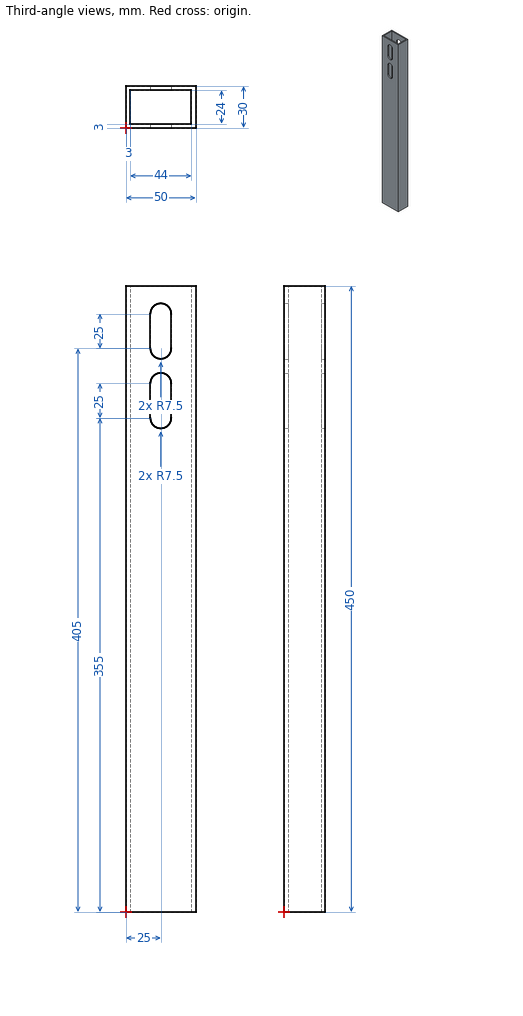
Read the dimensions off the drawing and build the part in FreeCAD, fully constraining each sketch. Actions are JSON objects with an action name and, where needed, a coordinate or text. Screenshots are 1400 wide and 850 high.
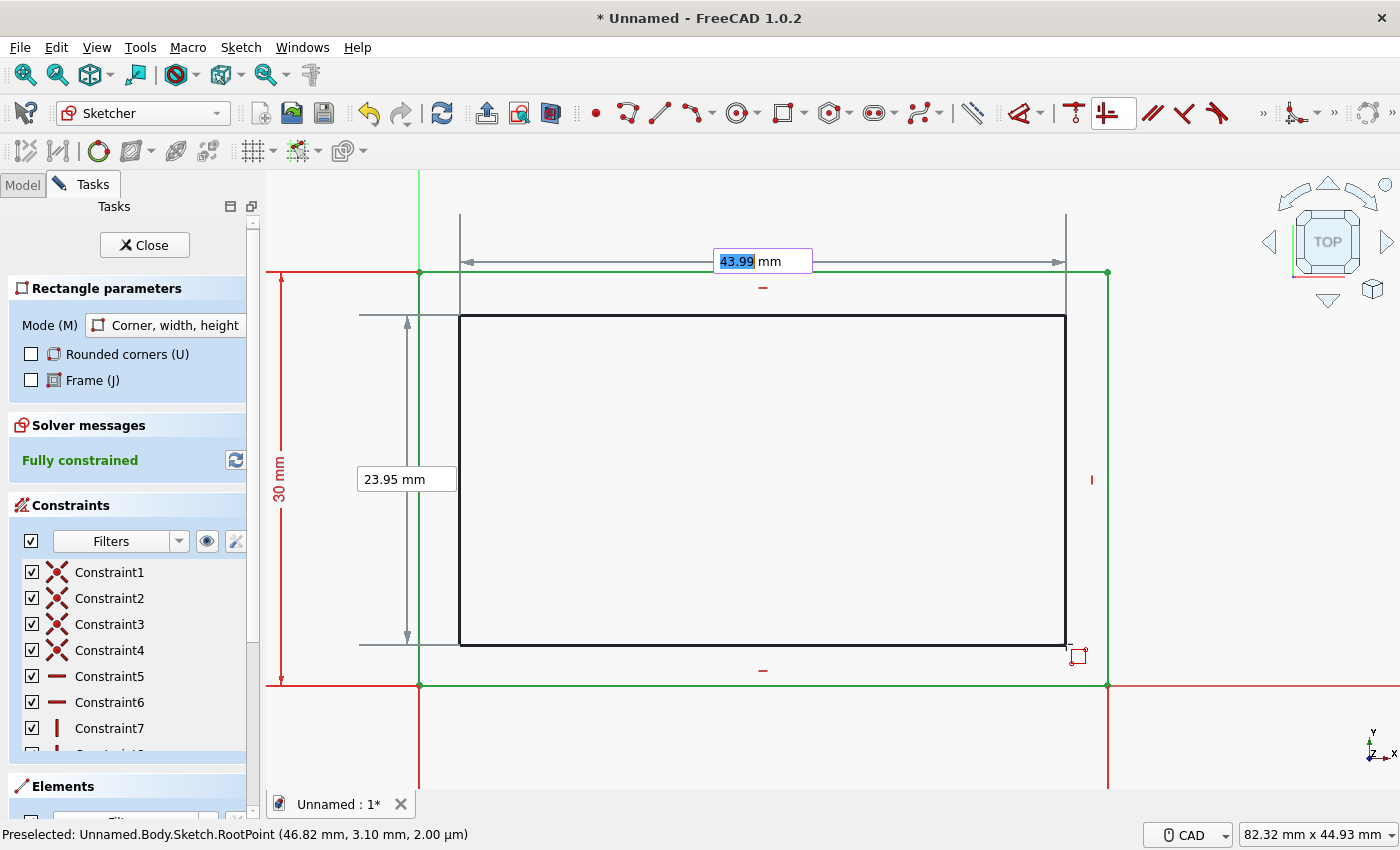
{"action": "type", "text": "44"}
{"action": "key", "text": "Tab"}
{"action": "type", "text": "24"}
{"action": "key", "text": "Return"}
{"action": "key", "text": "Escape"}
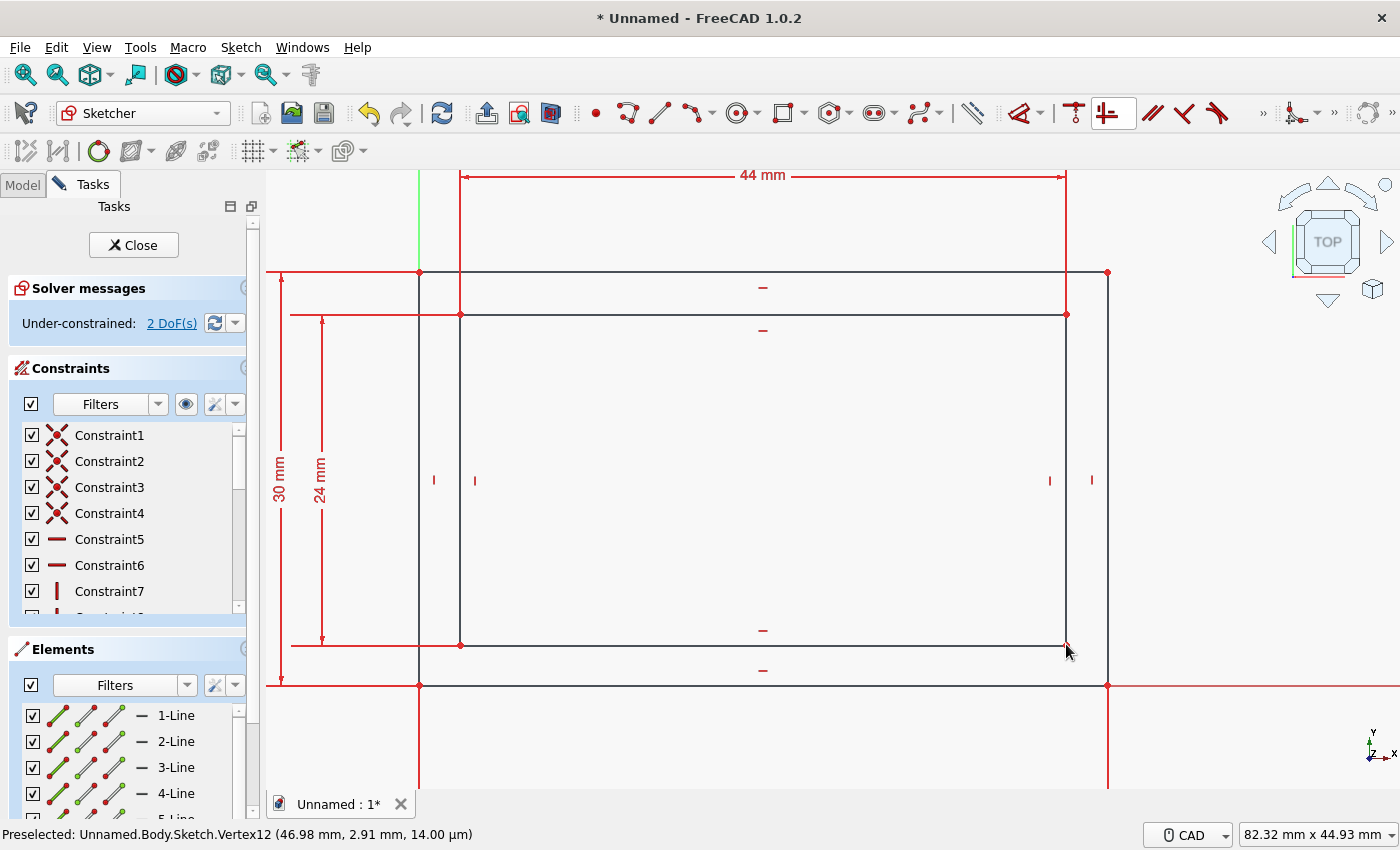
{"action": "left_click", "coordinate": [460, 315]}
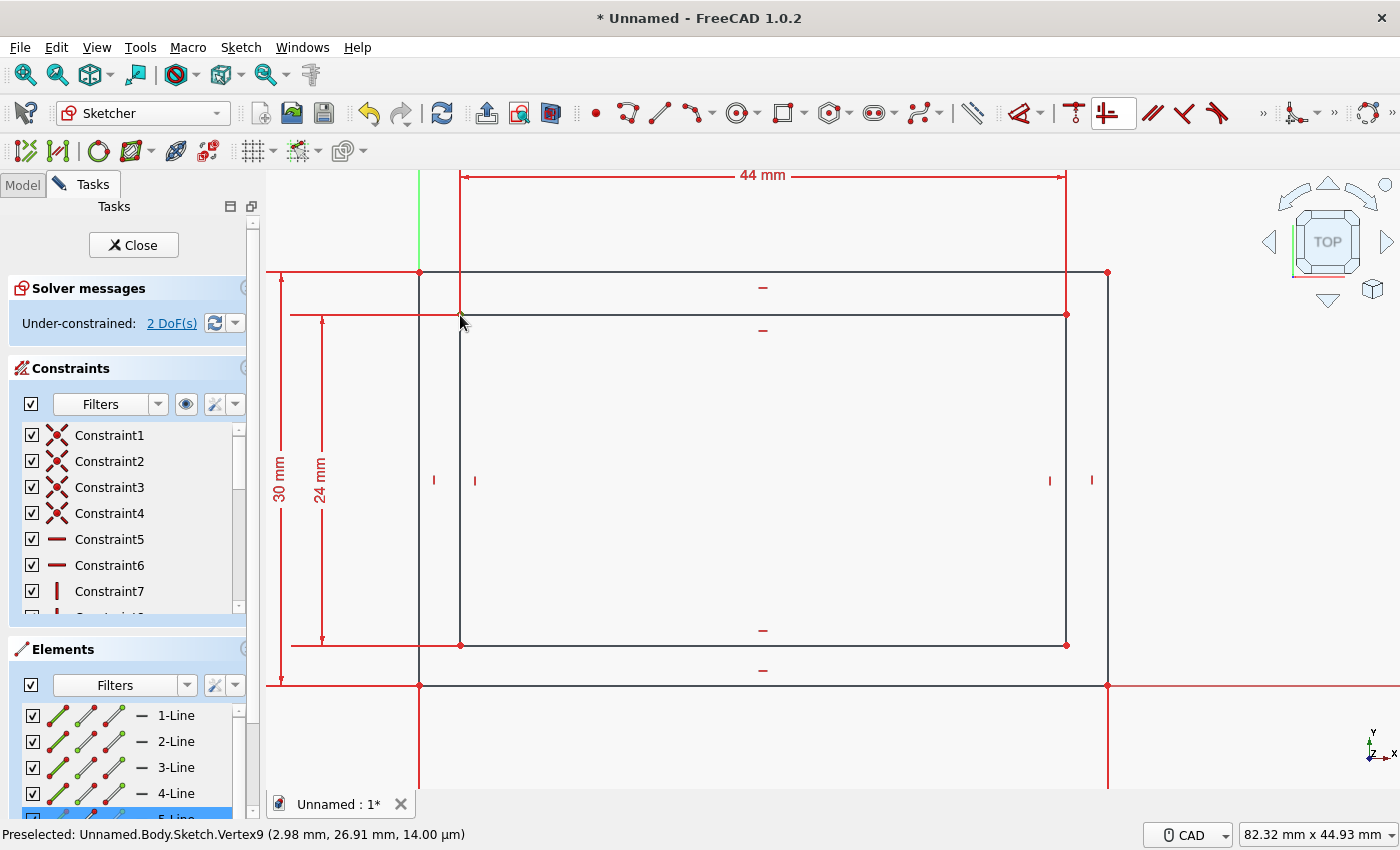
{"action": "key", "text": "l"}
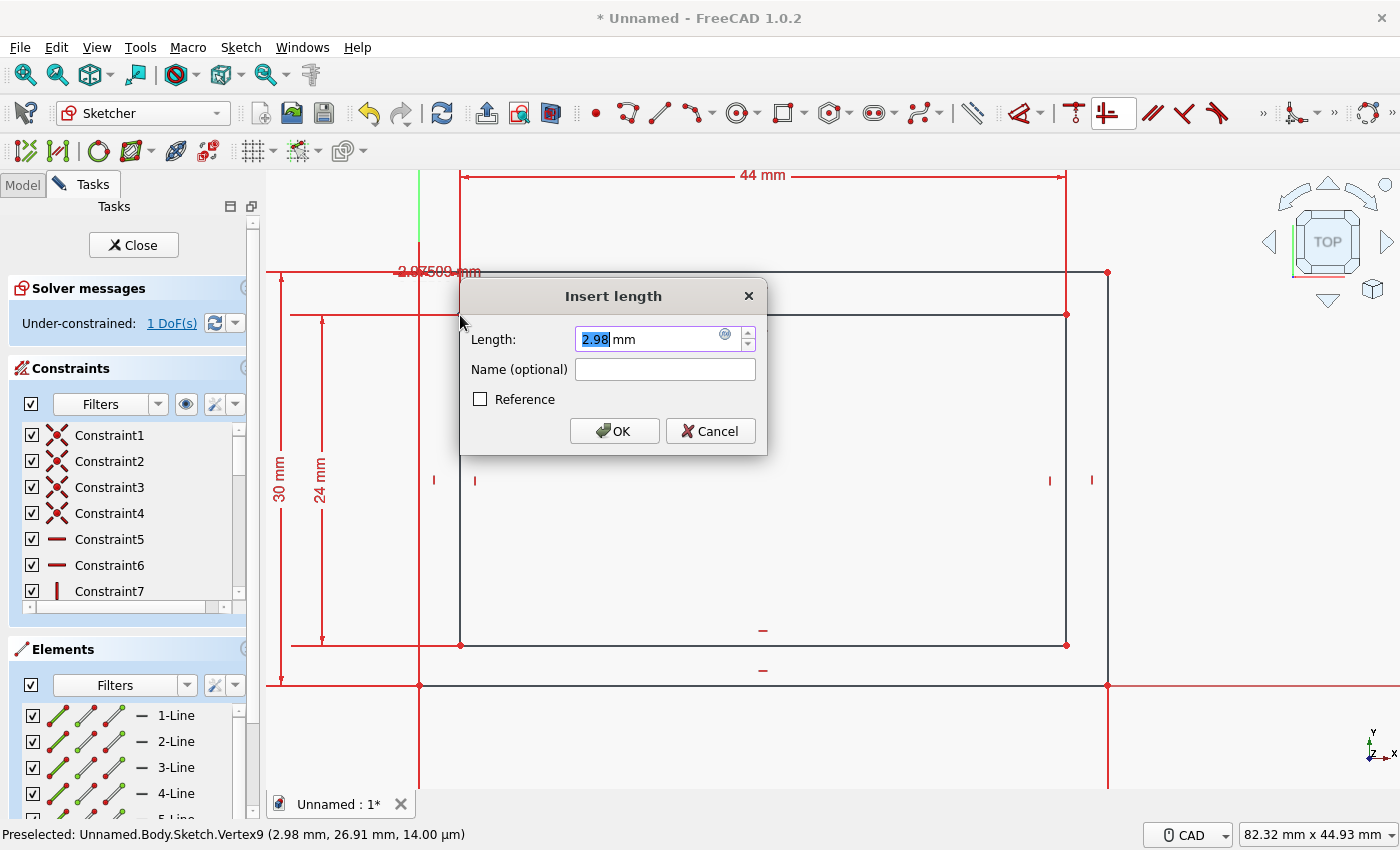
{"action": "type", "text": "3"}
{"action": "key", "text": "Return"}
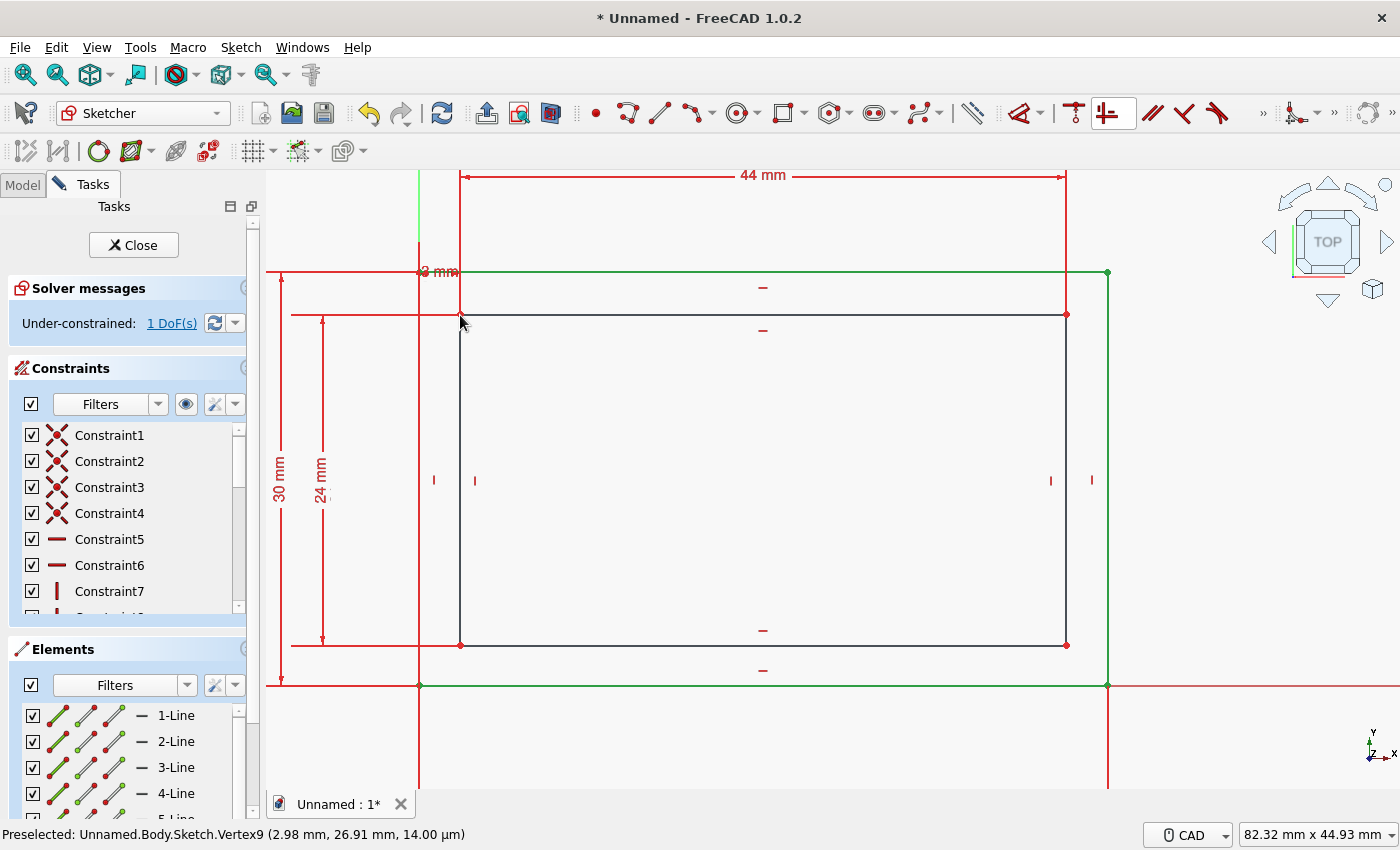
{"action": "left_click", "coordinate": [460, 646]}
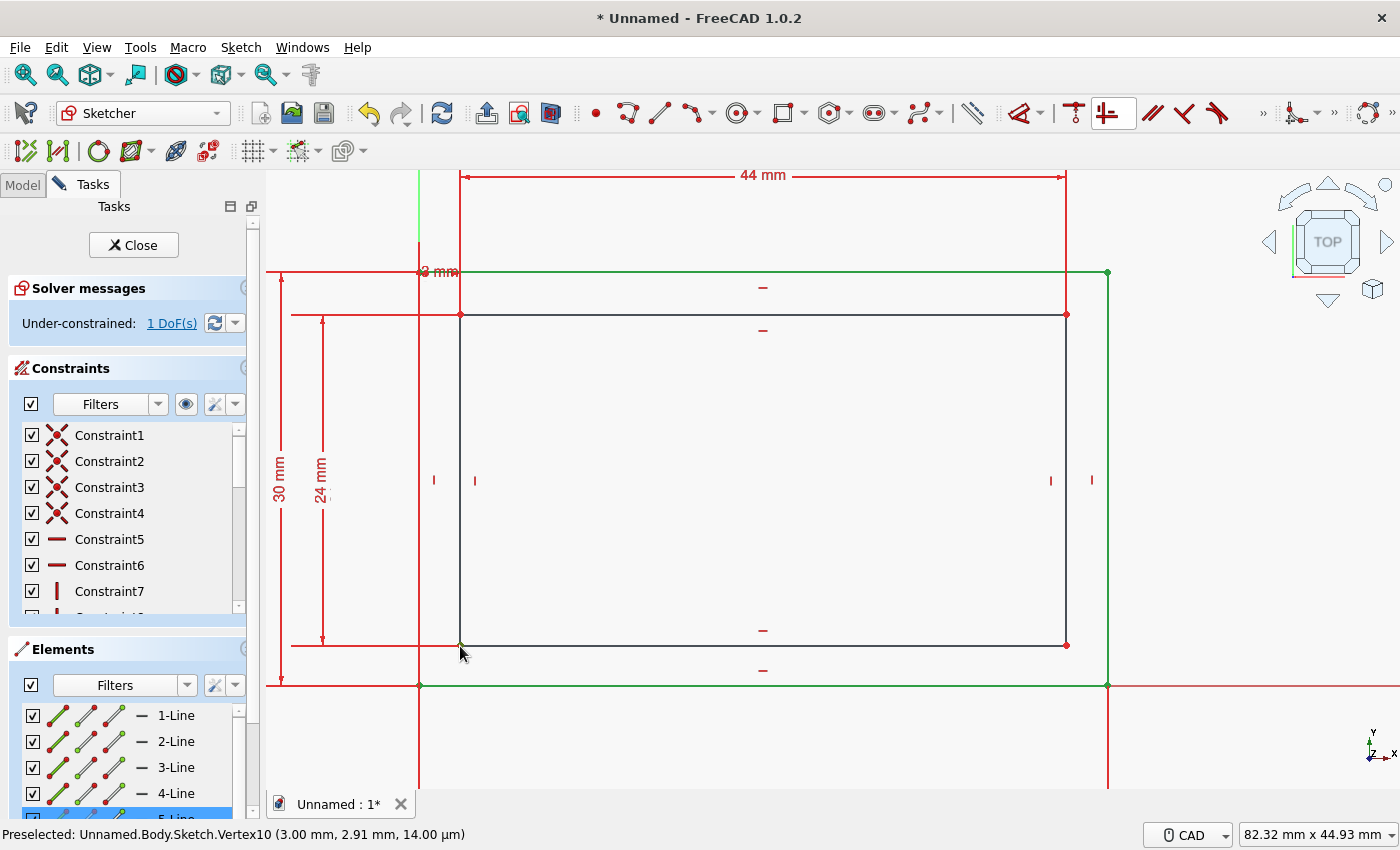
{"action": "key", "text": "i"}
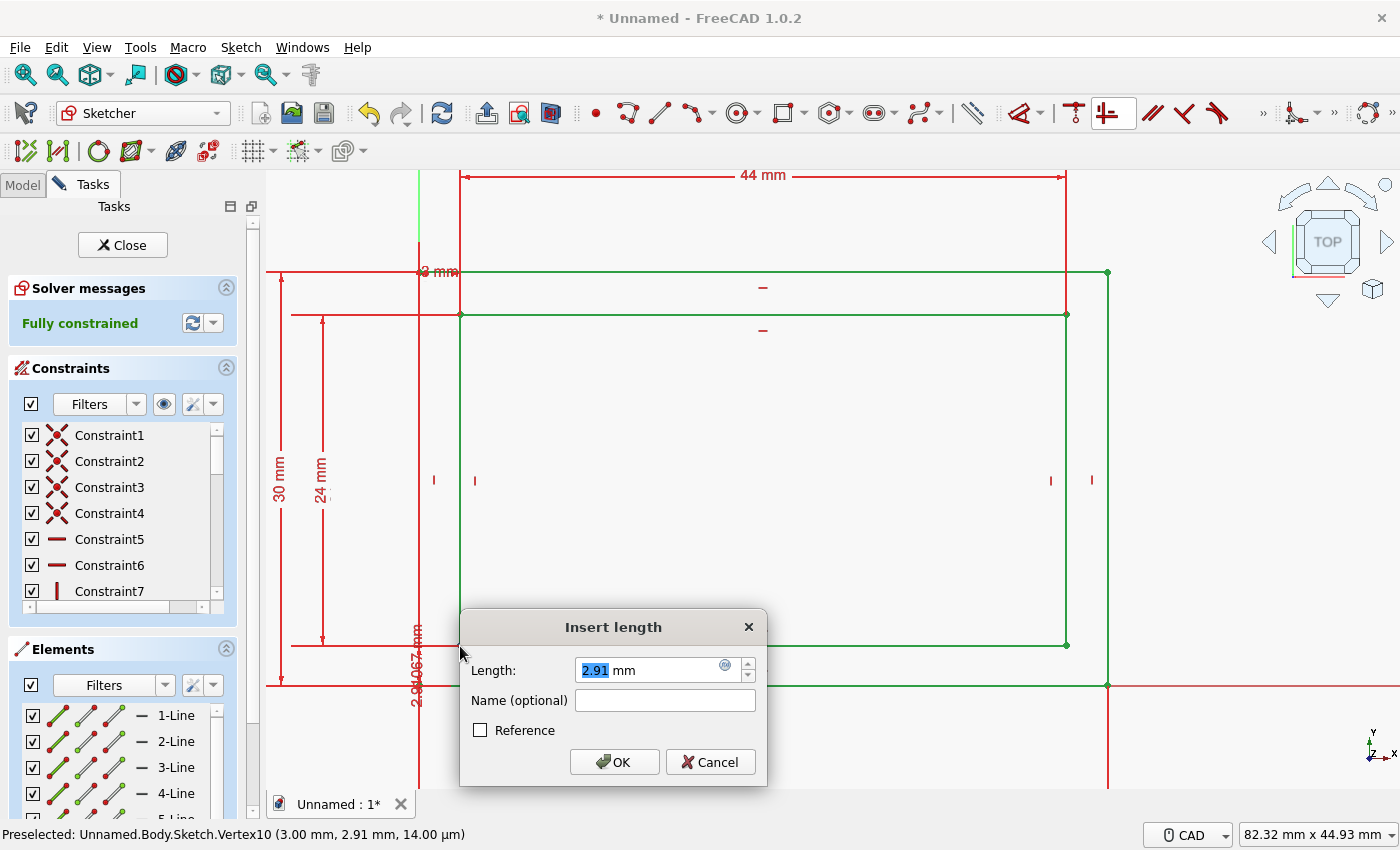
{"action": "type", "text": "3"}
{"action": "key", "text": "Return"}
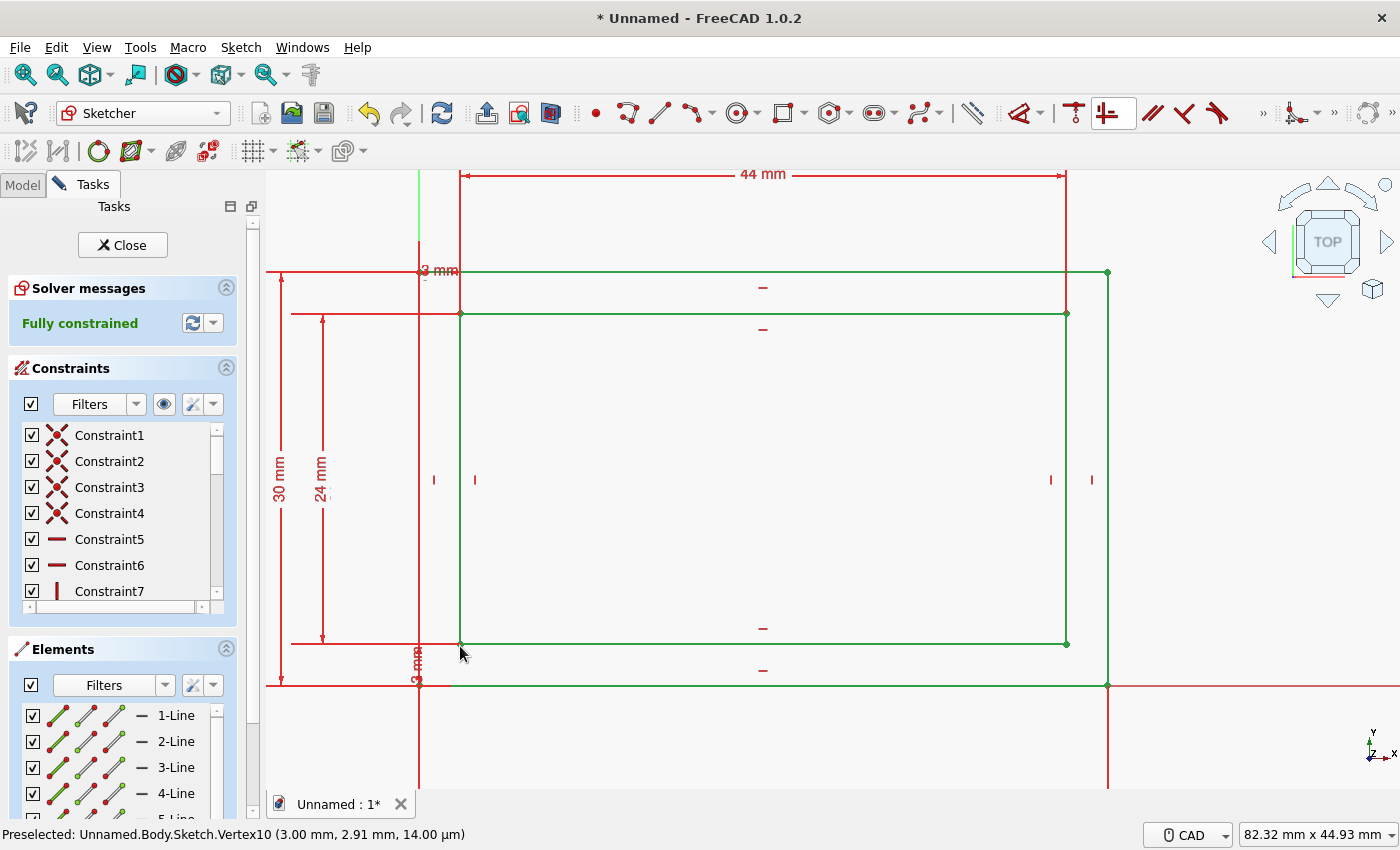
{"action": "left_click", "coordinate": [123, 245]}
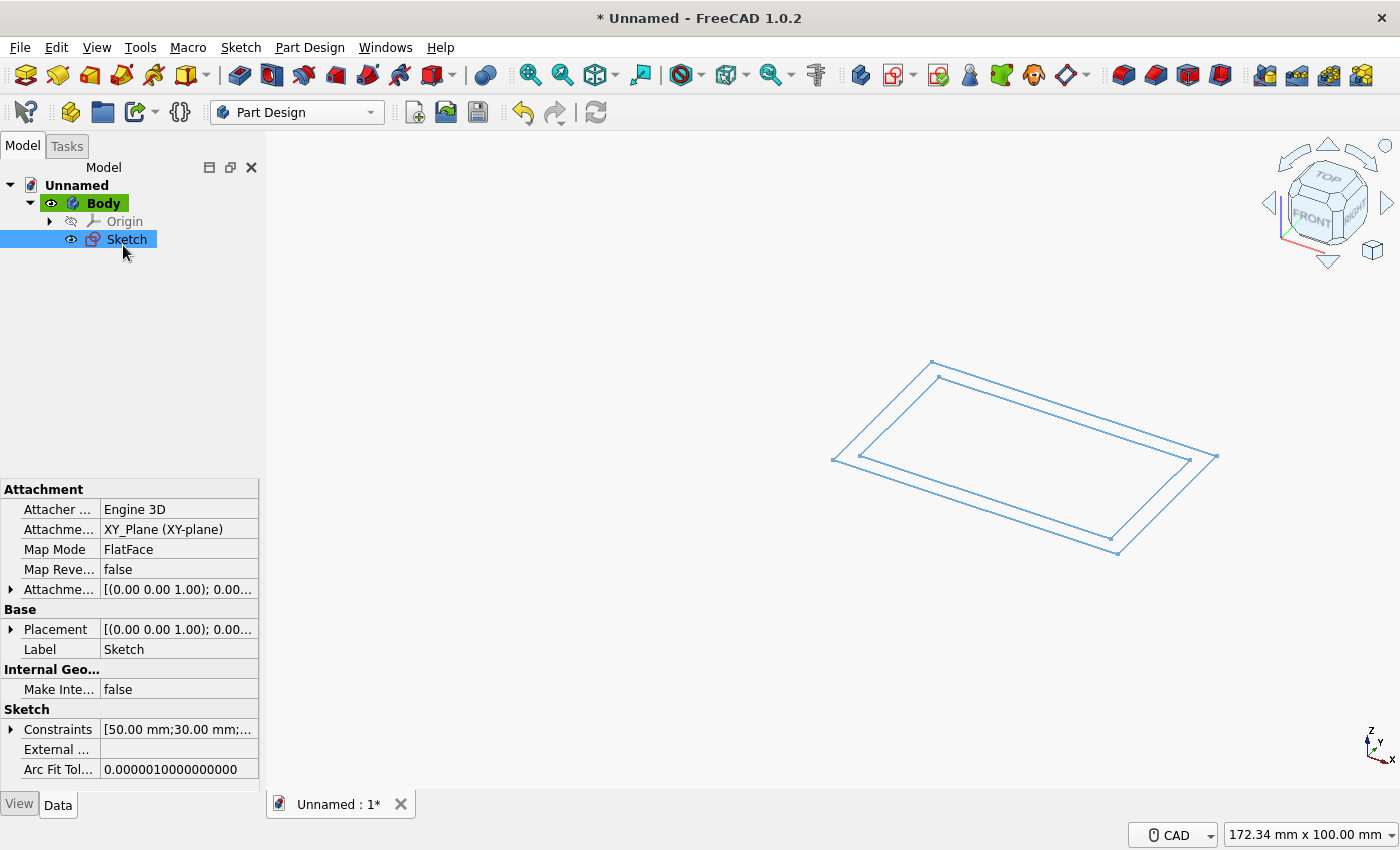
{"action": "left_click", "coordinate": [26, 76]}